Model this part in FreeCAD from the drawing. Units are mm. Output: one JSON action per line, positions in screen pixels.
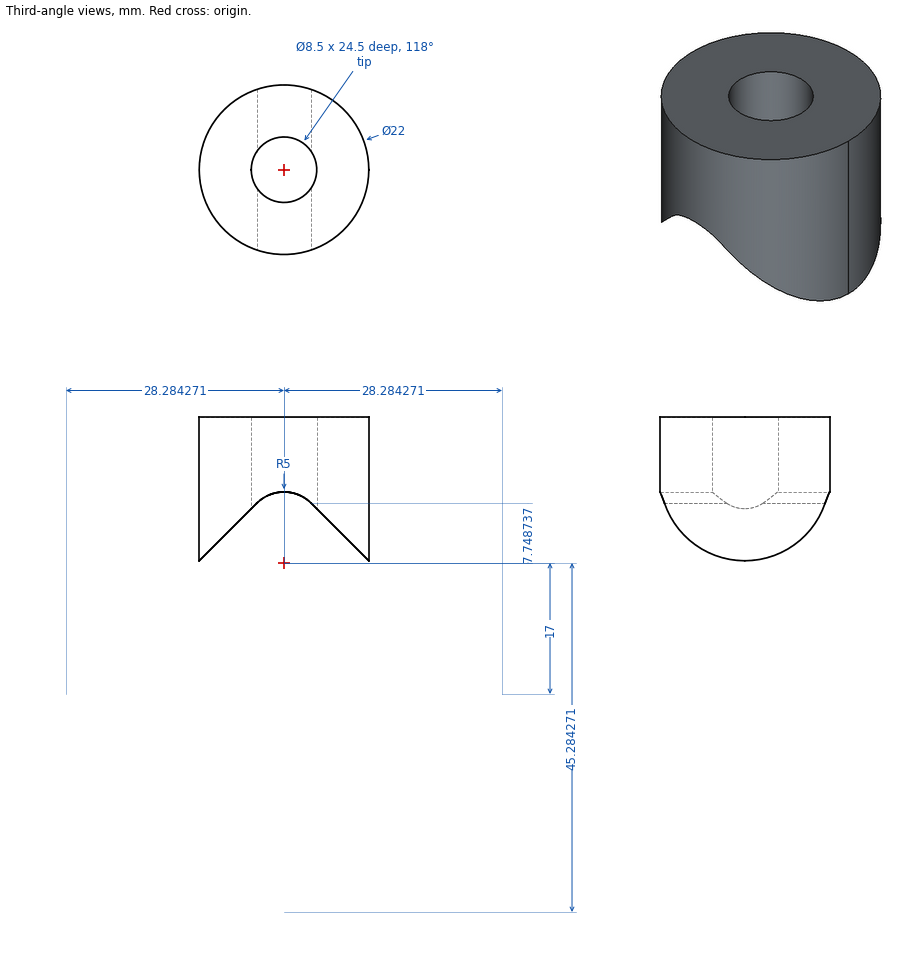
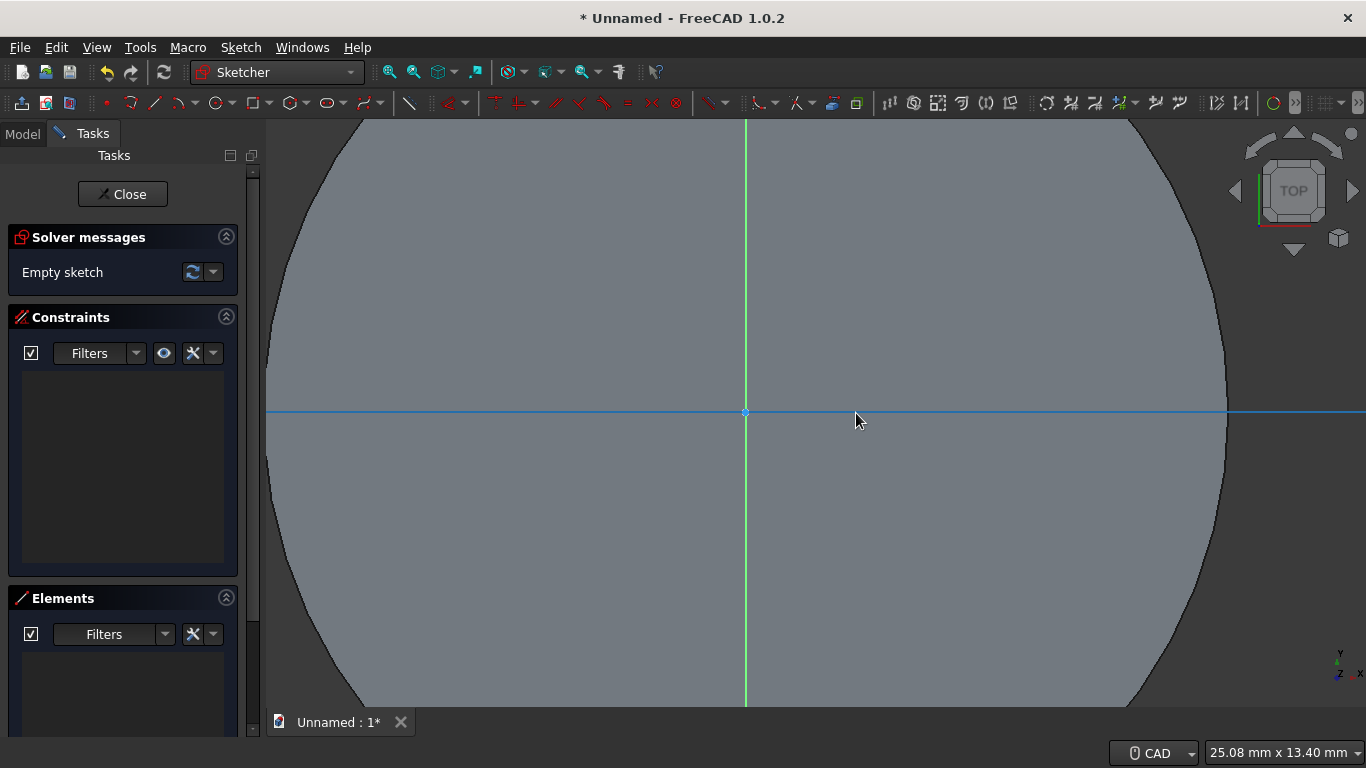
{"action": "key", "text": "g c"}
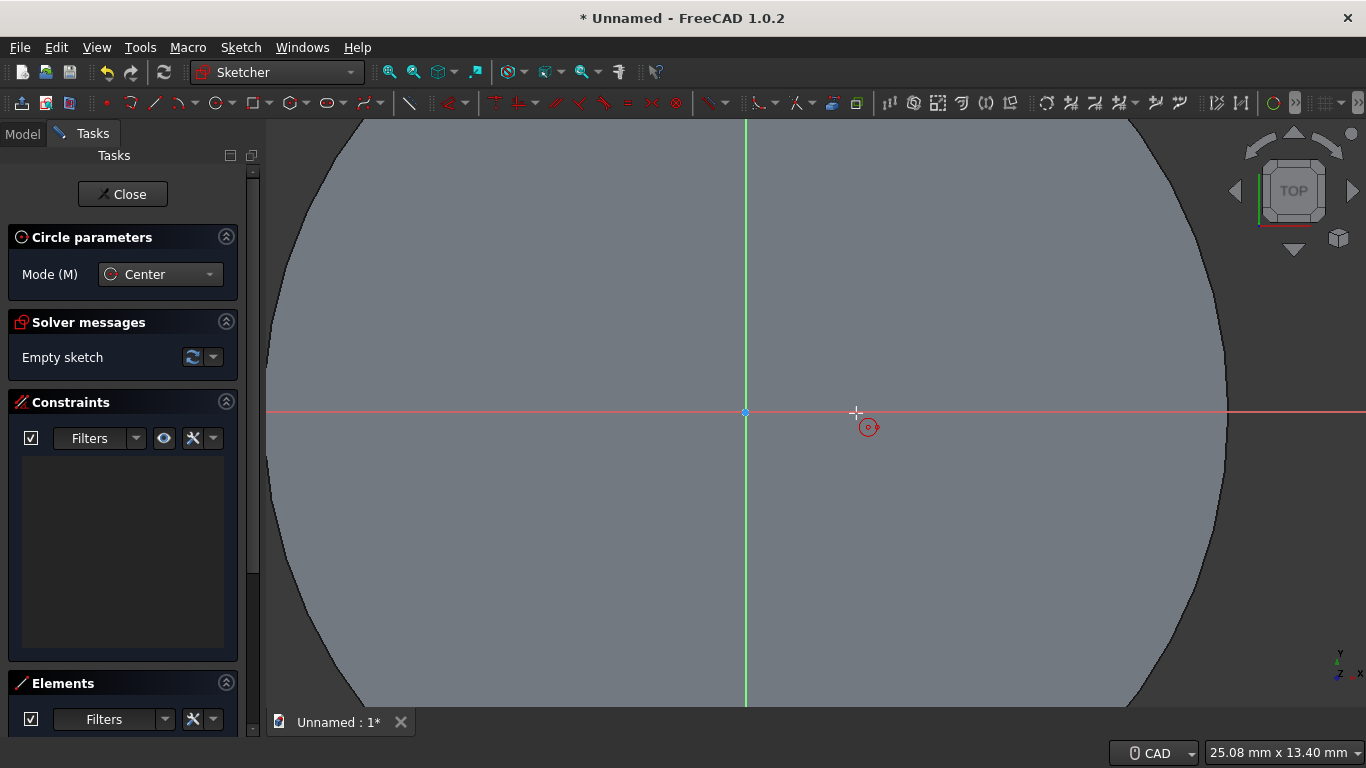
{"action": "left_click", "coordinate": [746, 412]}
{"action": "left_click", "coordinate": [878, 280]}
{"action": "key", "text": "Escape"}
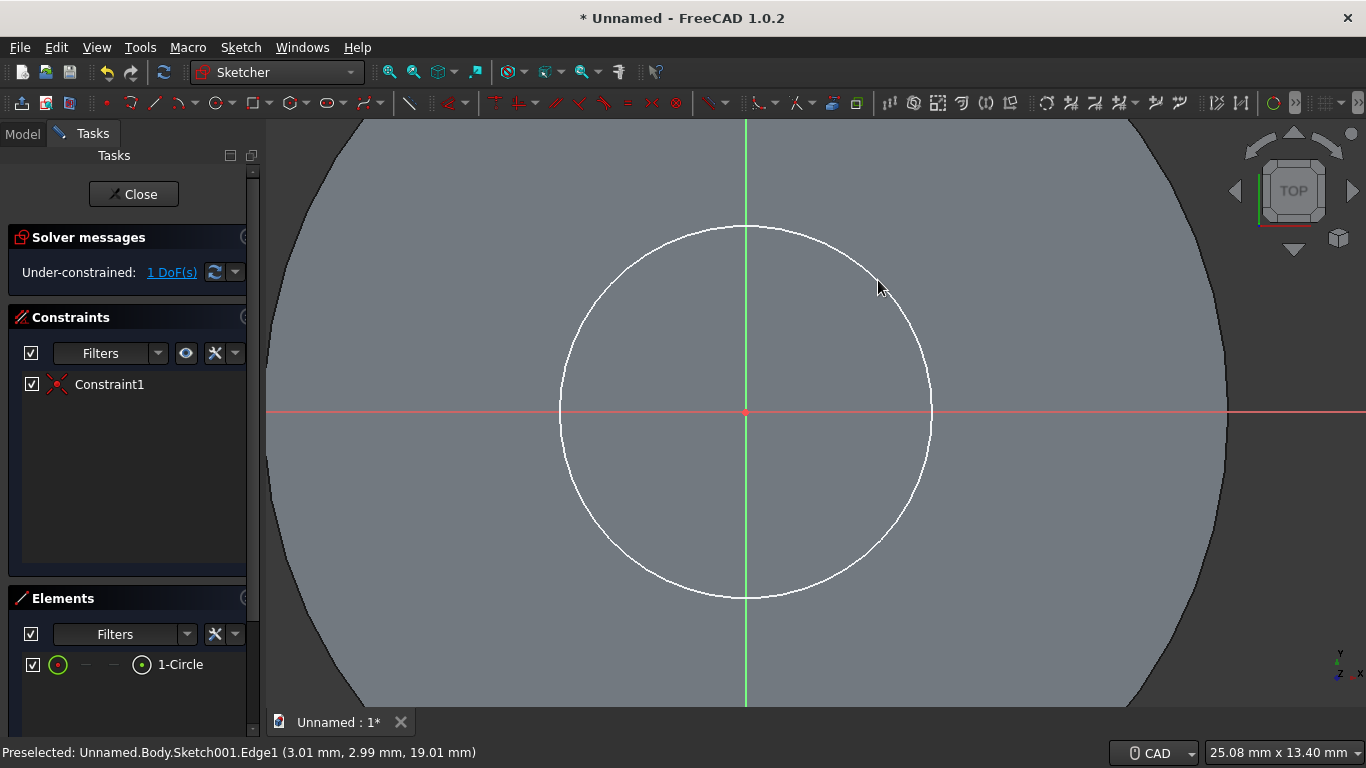
{"action": "key", "text": "d"}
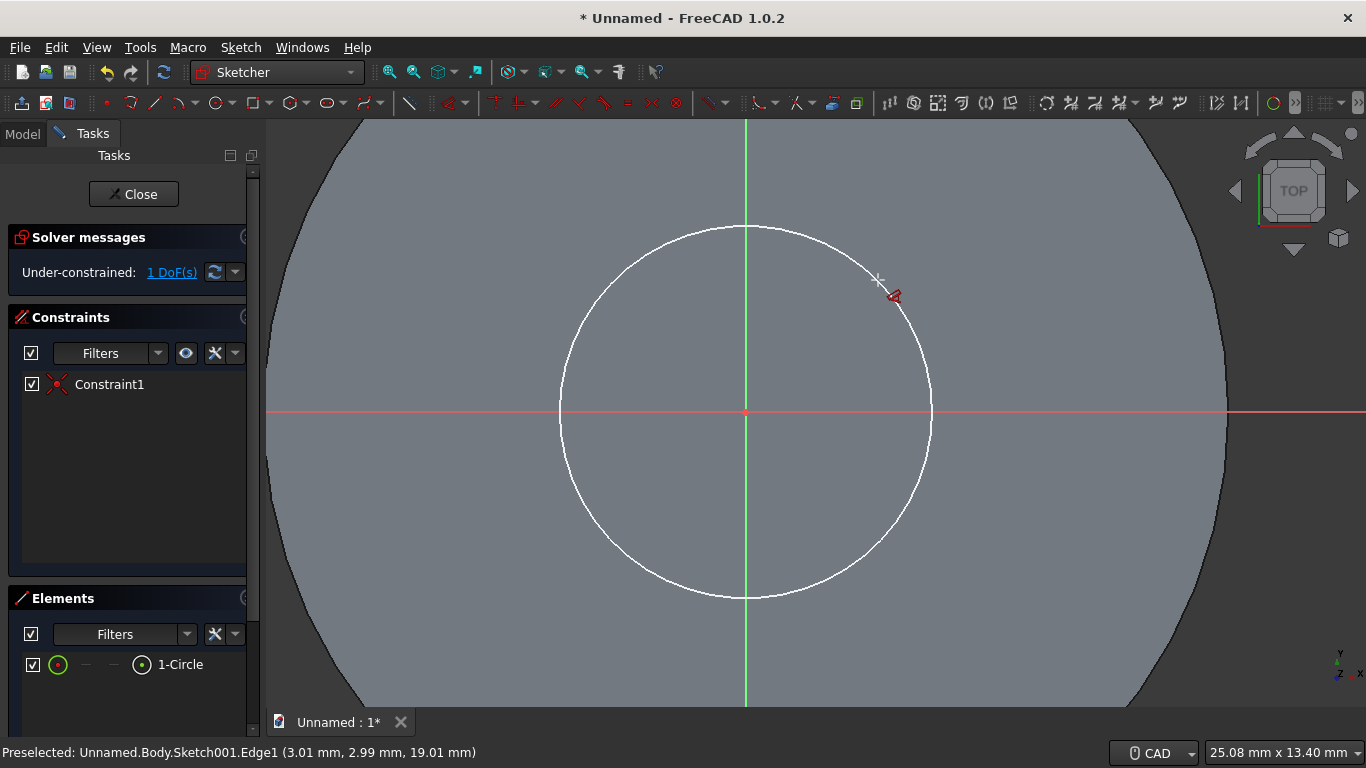
{"action": "left_click", "coordinate": [877, 280]}
{"action": "left_click", "coordinate": [900, 257]}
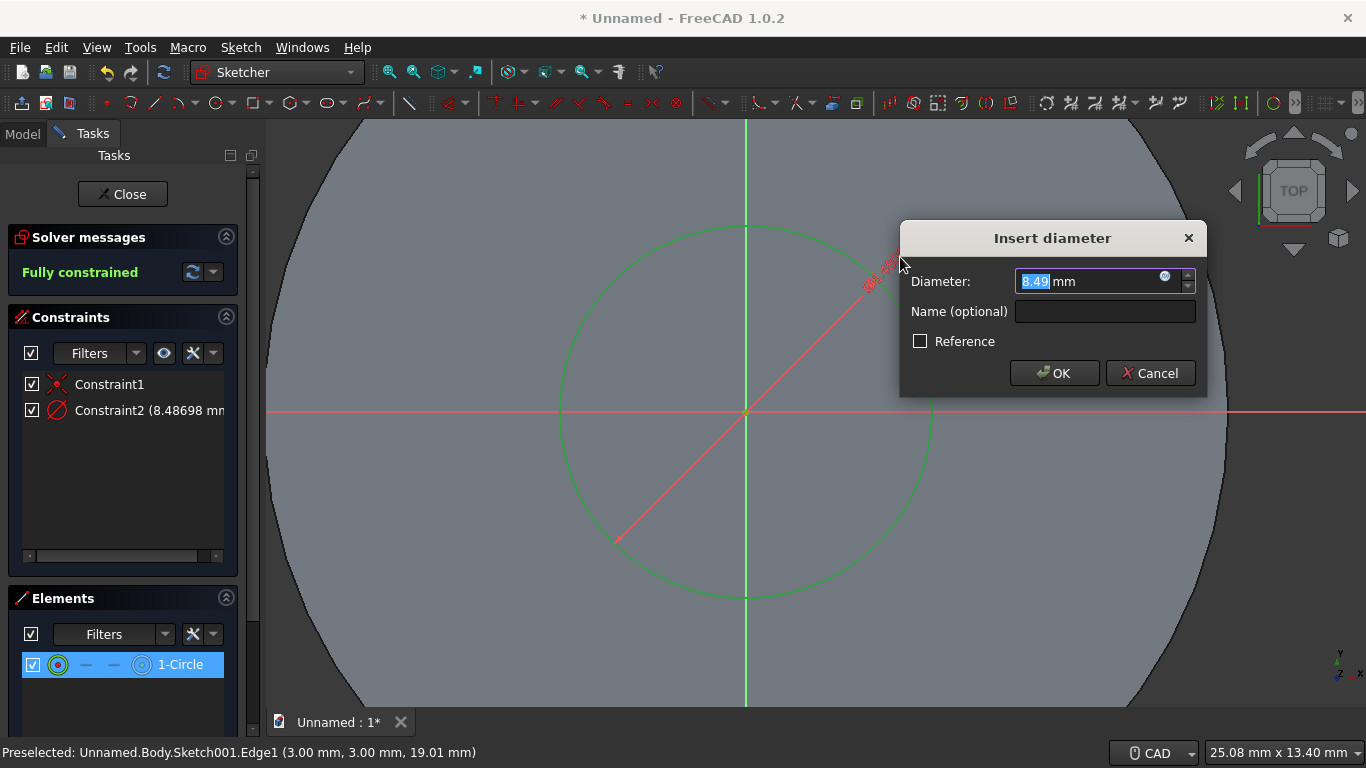
{"action": "type", "text": "8.5"}
{"action": "key", "text": "Return"}
{"action": "key", "text": "Escape"}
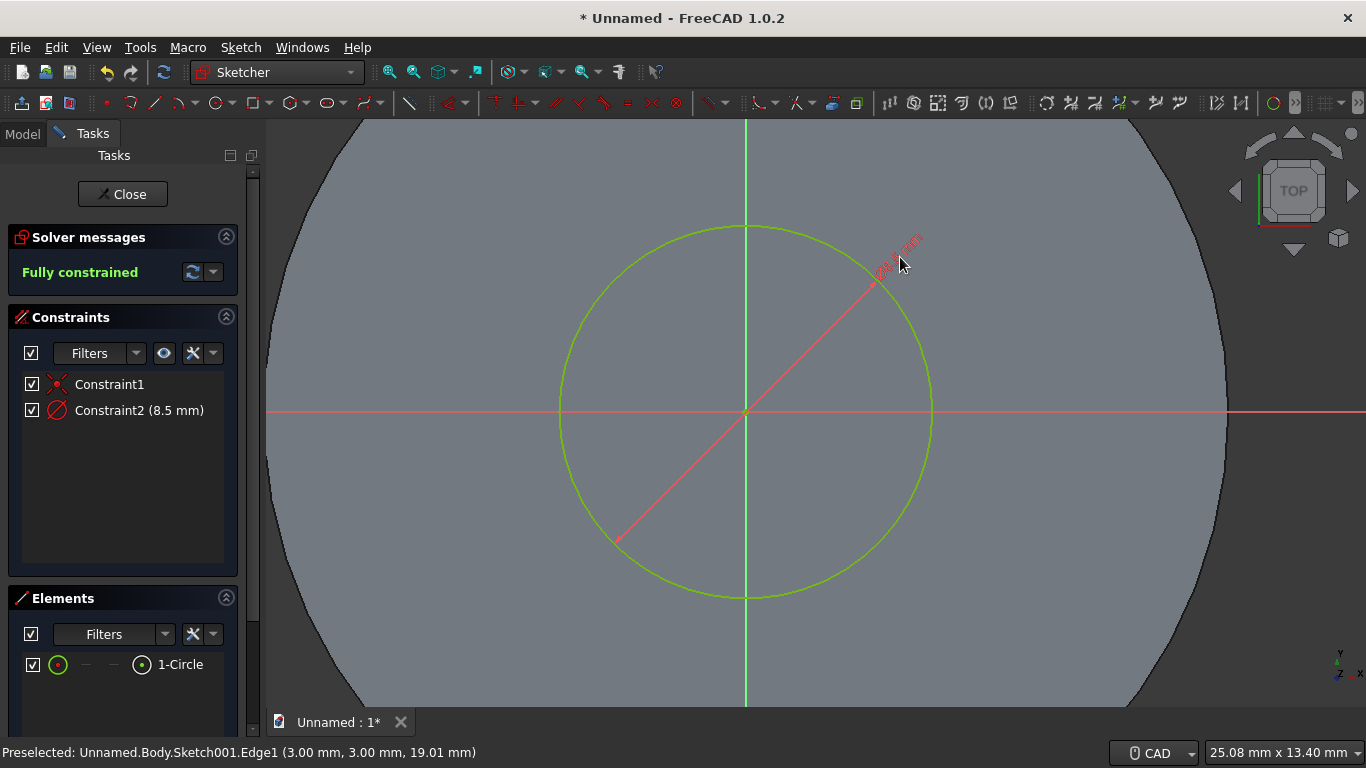
{"action": "left_click", "coordinate": [123, 194]}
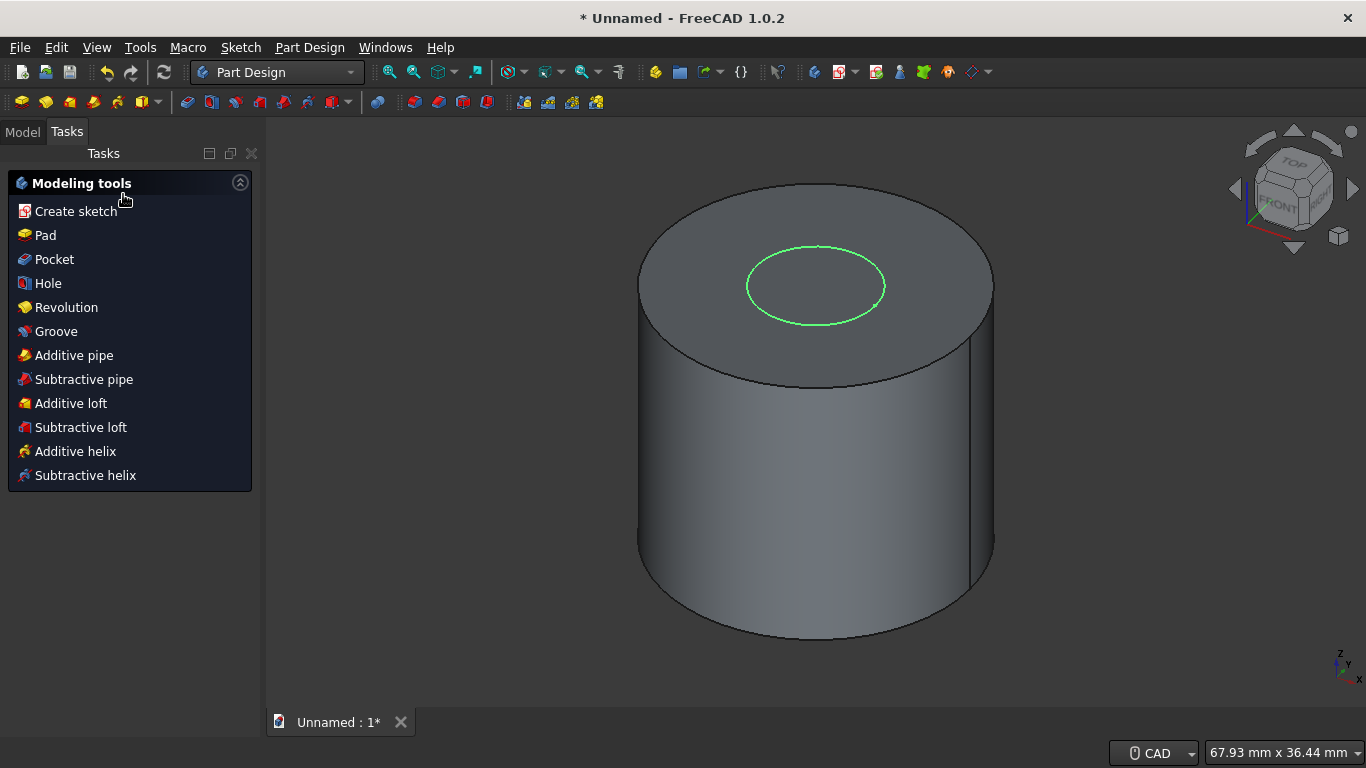
{"action": "left_click", "coordinate": [212, 102]}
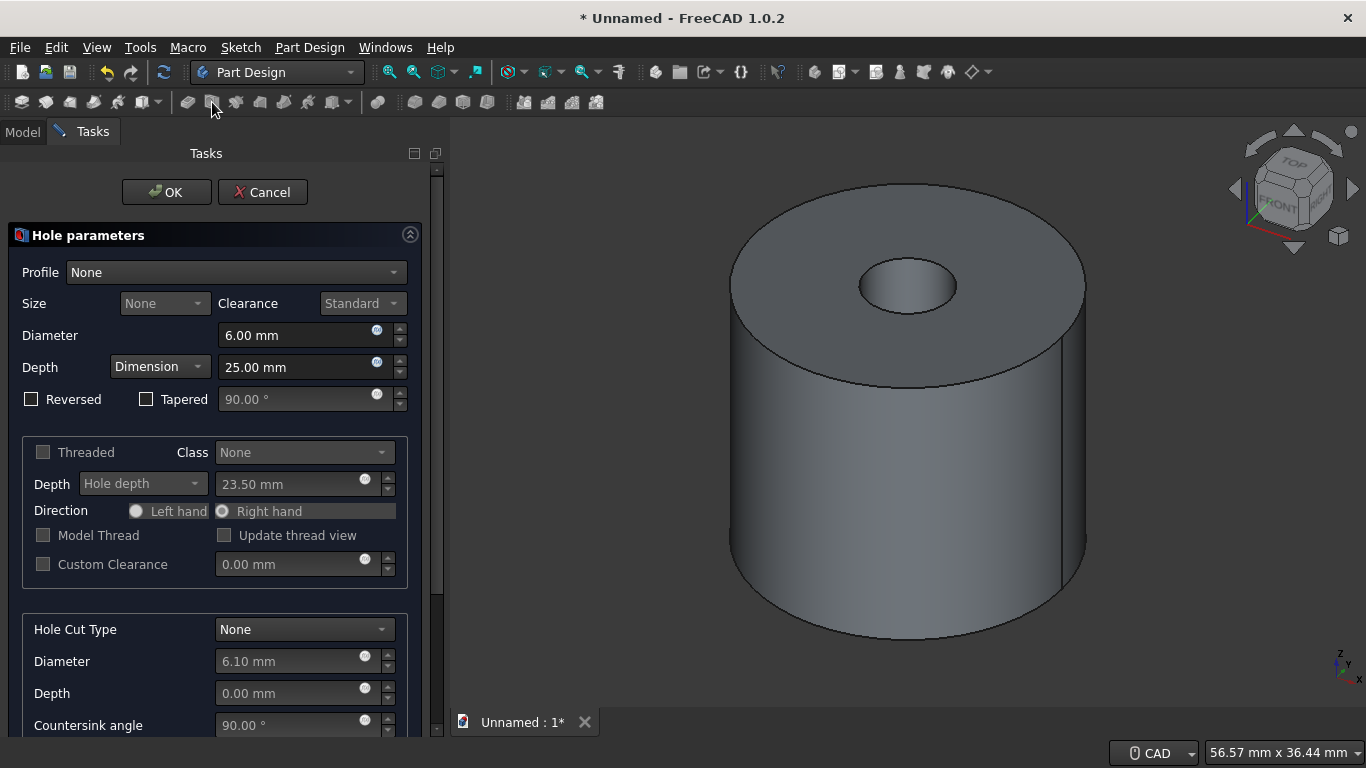
{"action": "triple_click", "coordinate": [305, 335]}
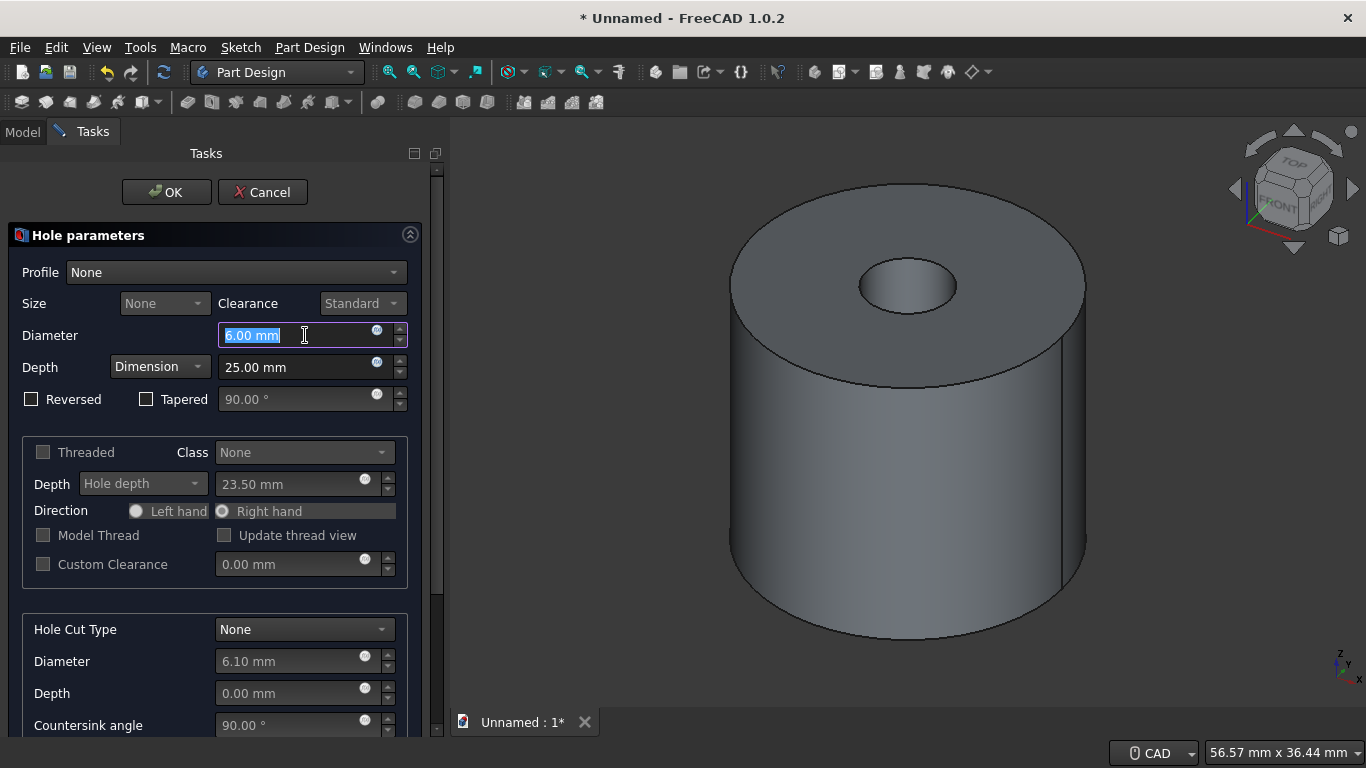
{"action": "type", "text": "8.5"}
{"action": "key", "text": "Tab"}